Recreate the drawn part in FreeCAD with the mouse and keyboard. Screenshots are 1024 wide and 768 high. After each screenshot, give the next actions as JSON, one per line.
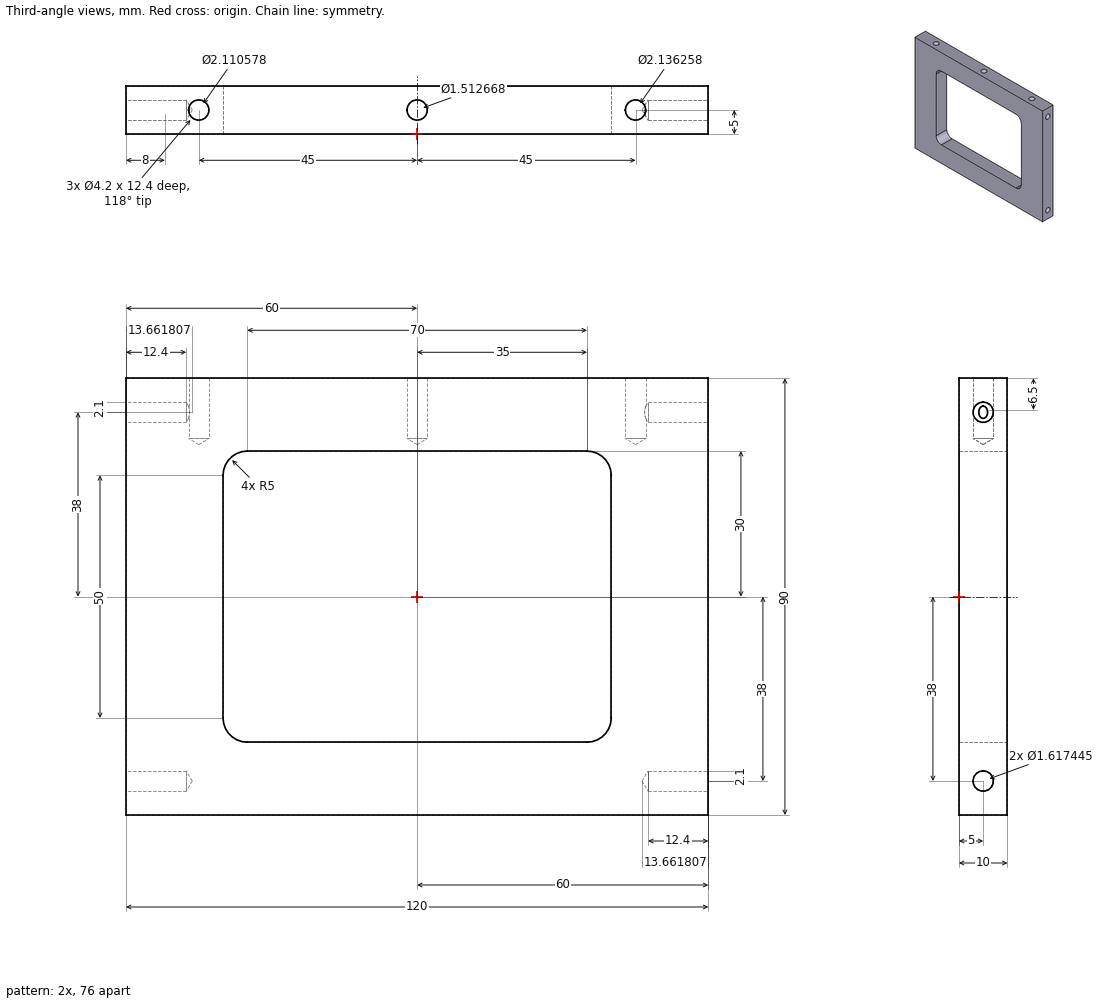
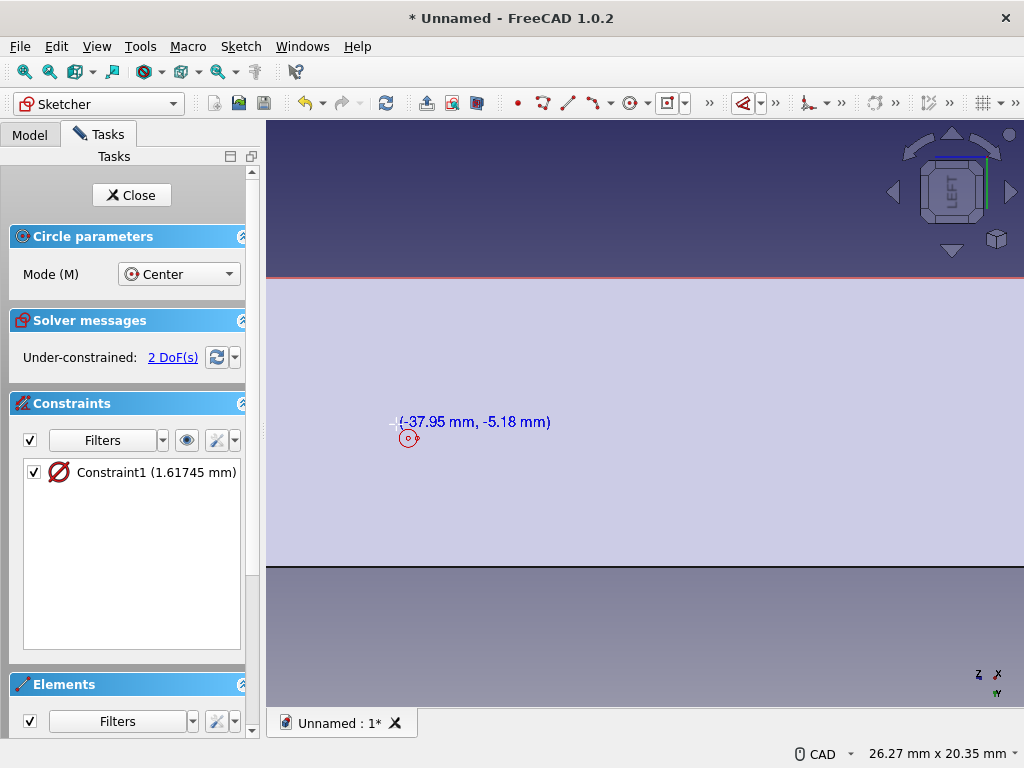
{"action": "scroll", "coordinate": [396, 424], "scroll_direction": "down", "scroll_amount": 9}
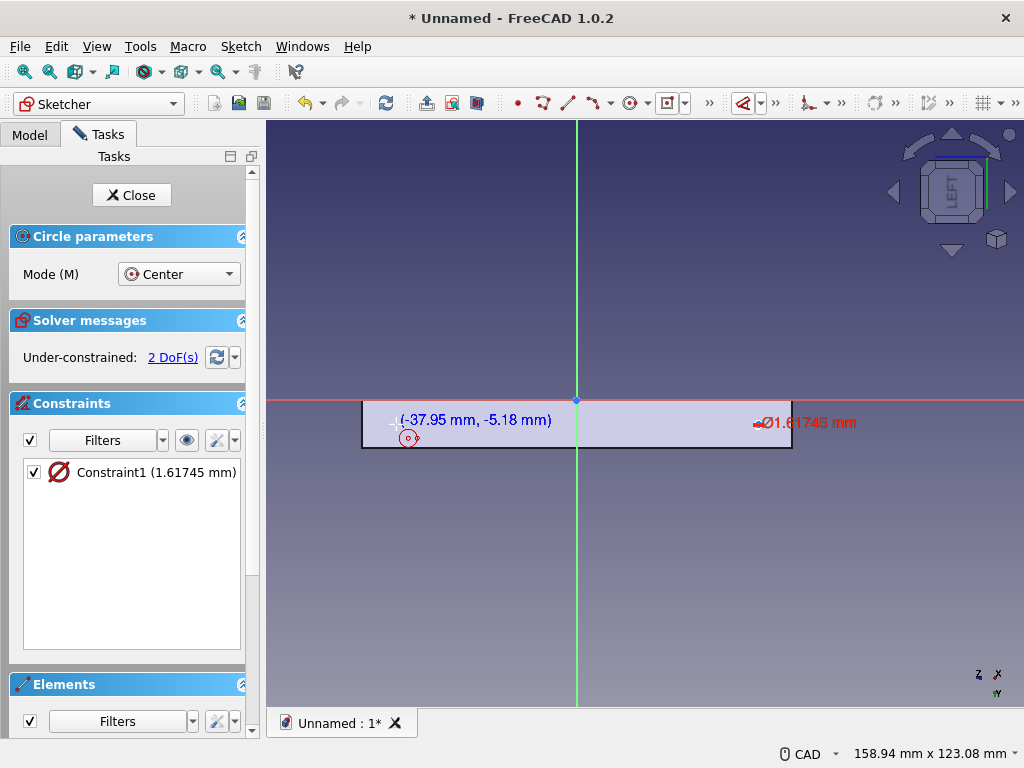
{"action": "left_click", "coordinate": [396, 424]}
{"action": "mouse_move", "coordinate": [398, 421]}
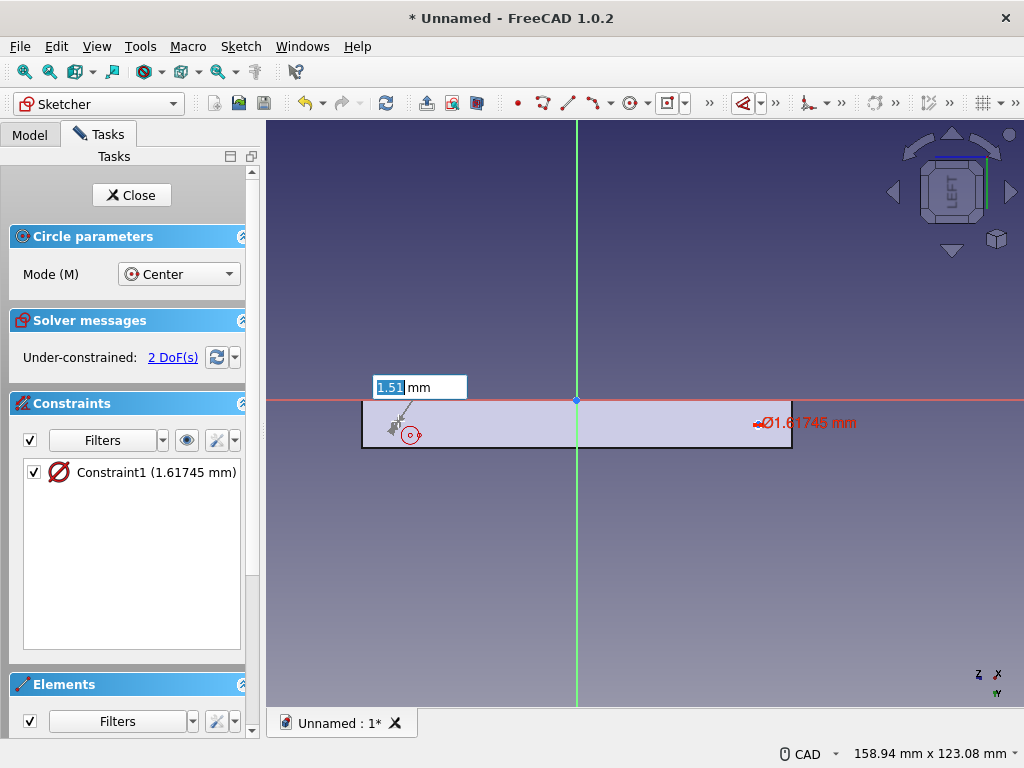
{"action": "type", "text": "1.617445"}
{"action": "key", "text": "Return"}
{"action": "key", "text": "Escape"}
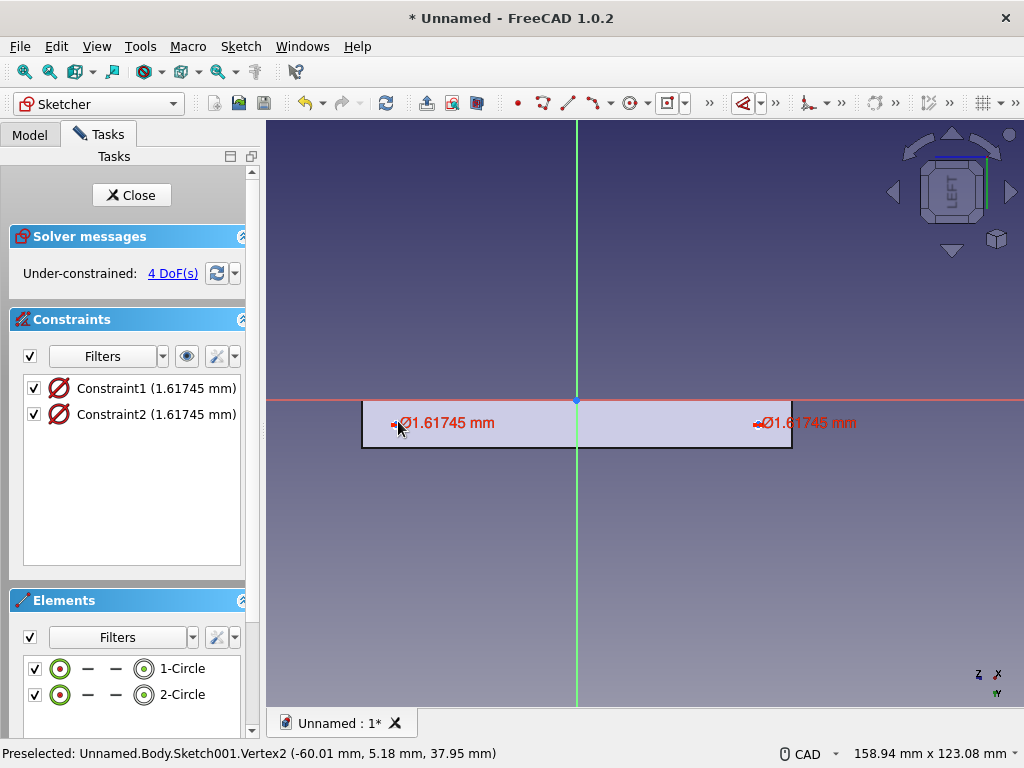
{"action": "left_click", "coordinate": [758, 425]}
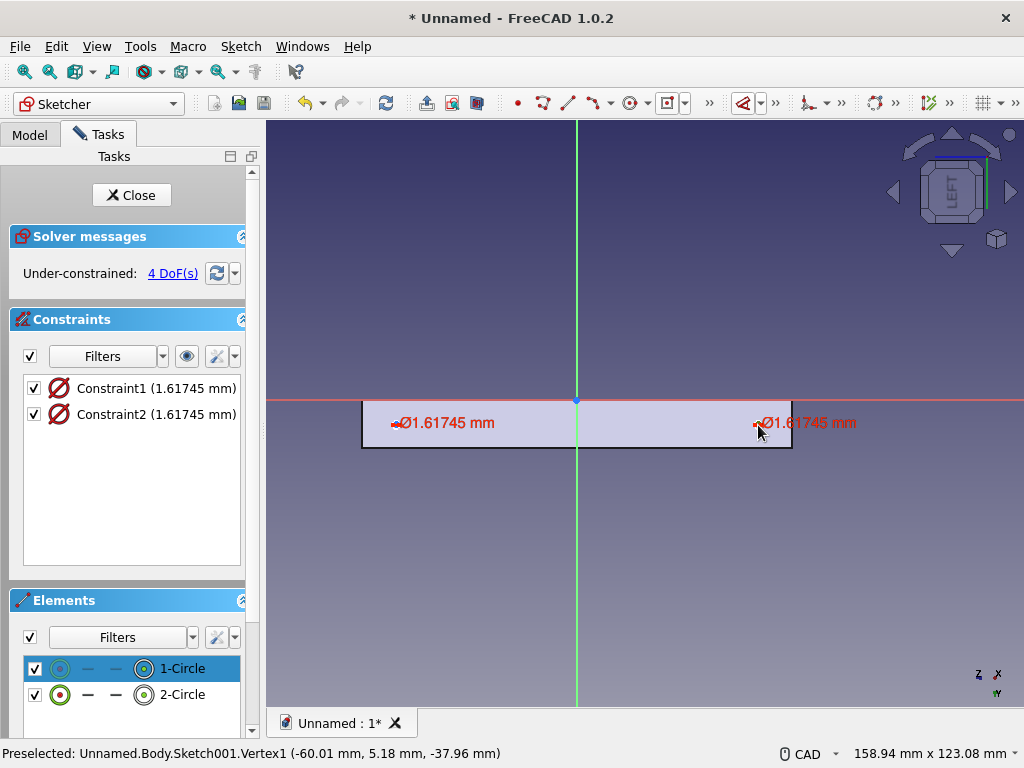
{"action": "left_click", "coordinate": [396, 425]}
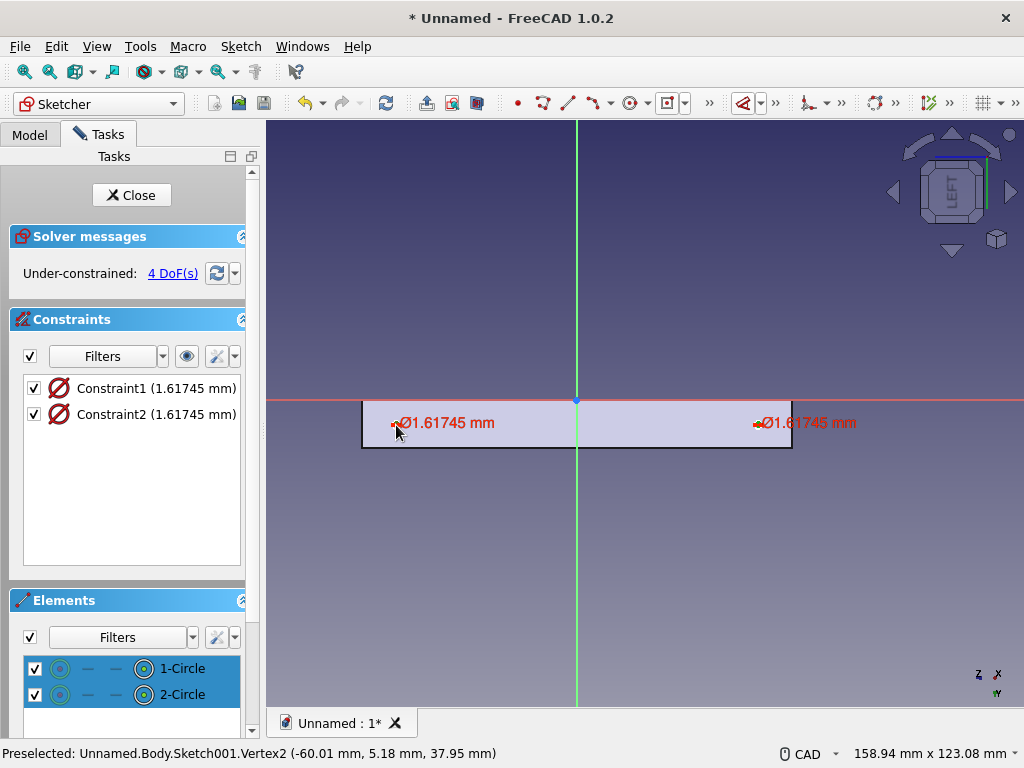
{"action": "left_click", "coordinate": [577, 641]}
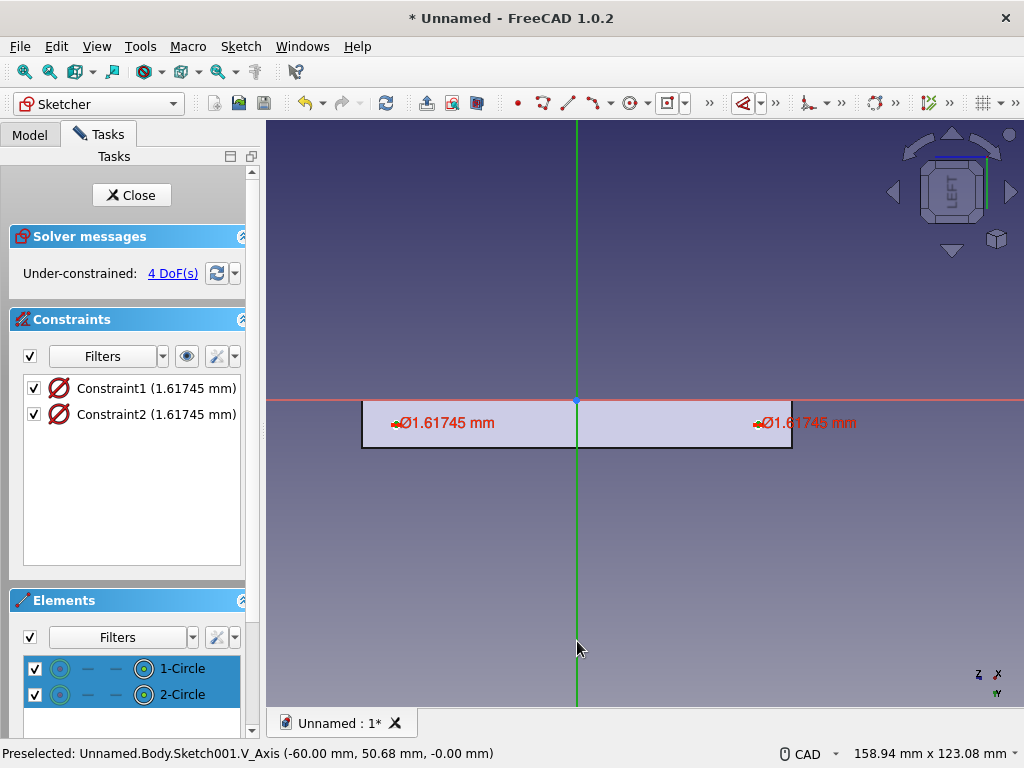
{"action": "key", "text": "s"}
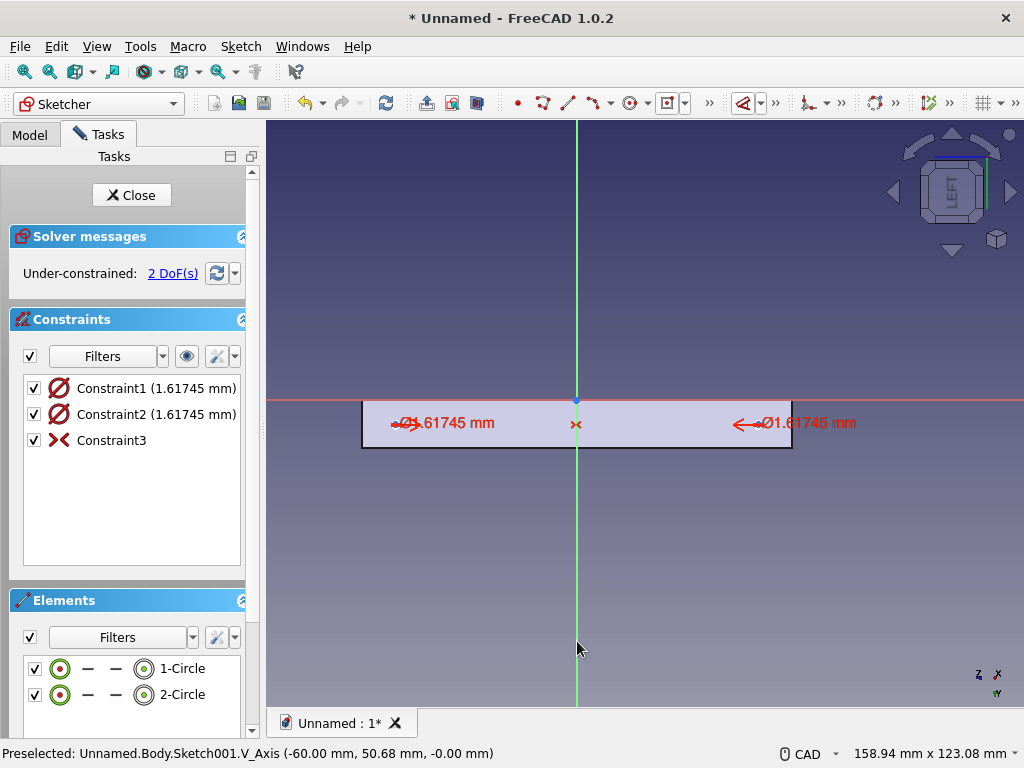
{"action": "left_click", "coordinate": [742, 104]}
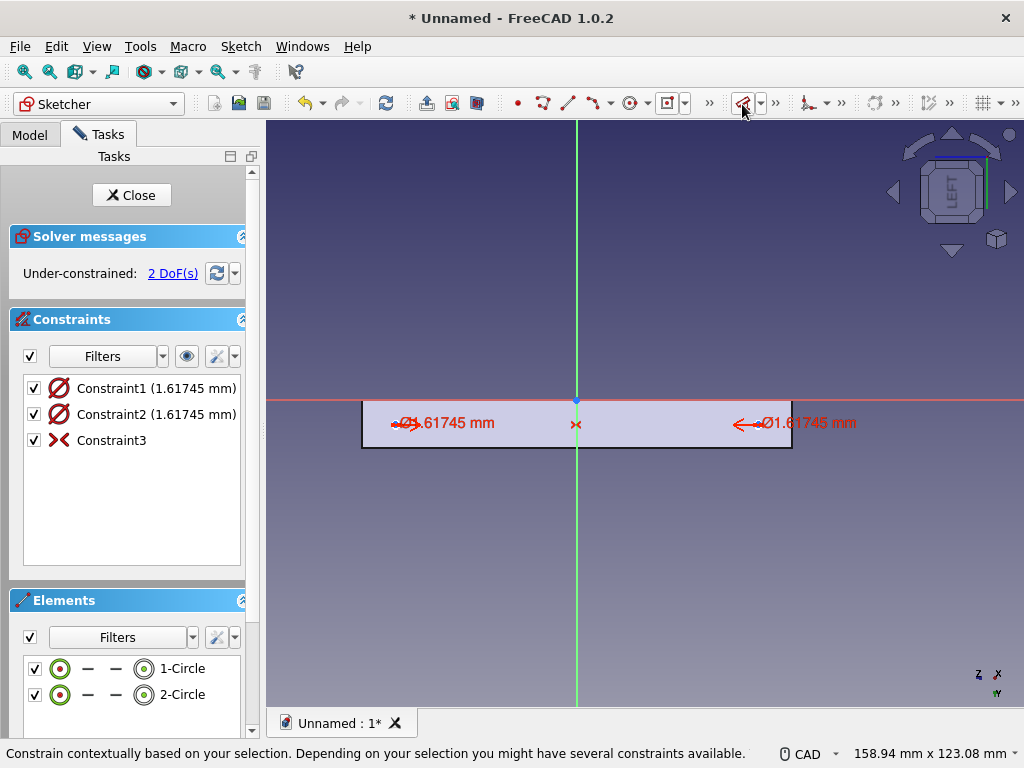
{"action": "scroll", "coordinate": [758, 425], "scroll_direction": "up", "scroll_amount": 3}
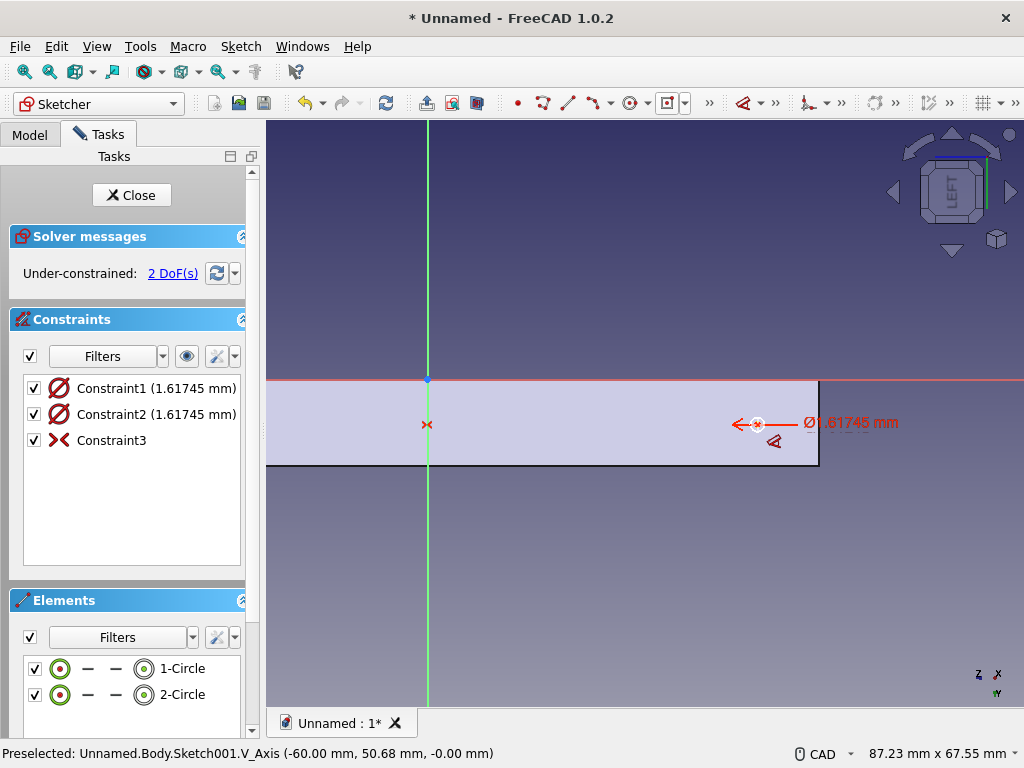
{"action": "left_click", "coordinate": [757, 425]}
{"action": "left_click", "coordinate": [791, 402]}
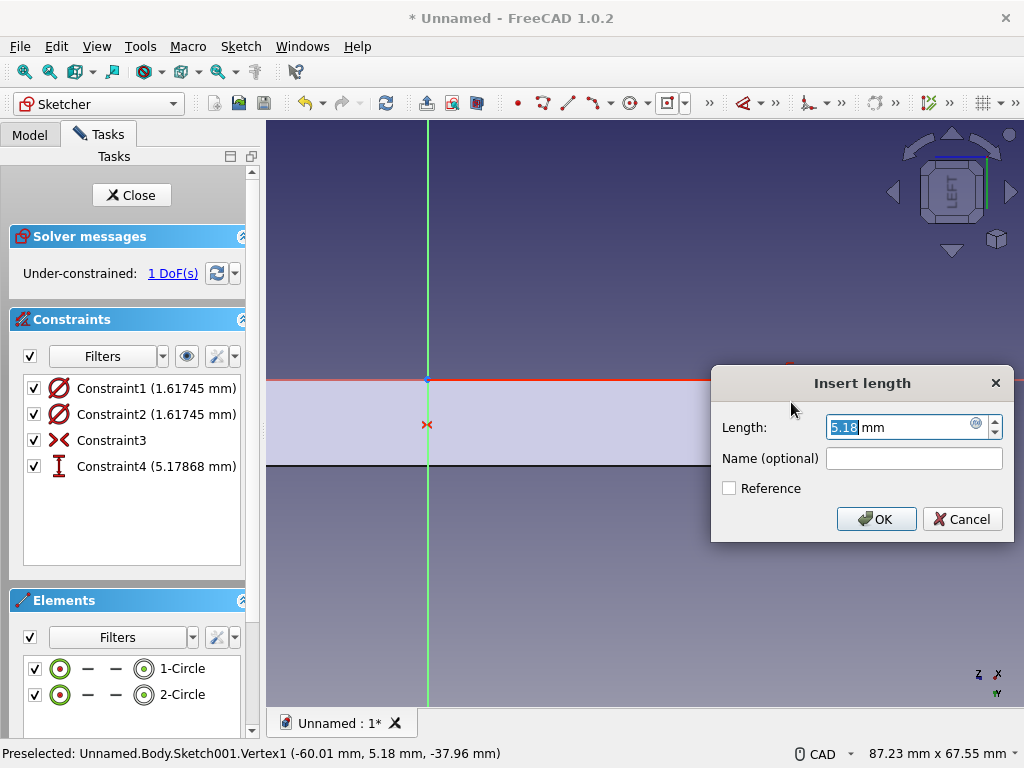
{"action": "type", "text": "5"}
{"action": "key", "text": "Return"}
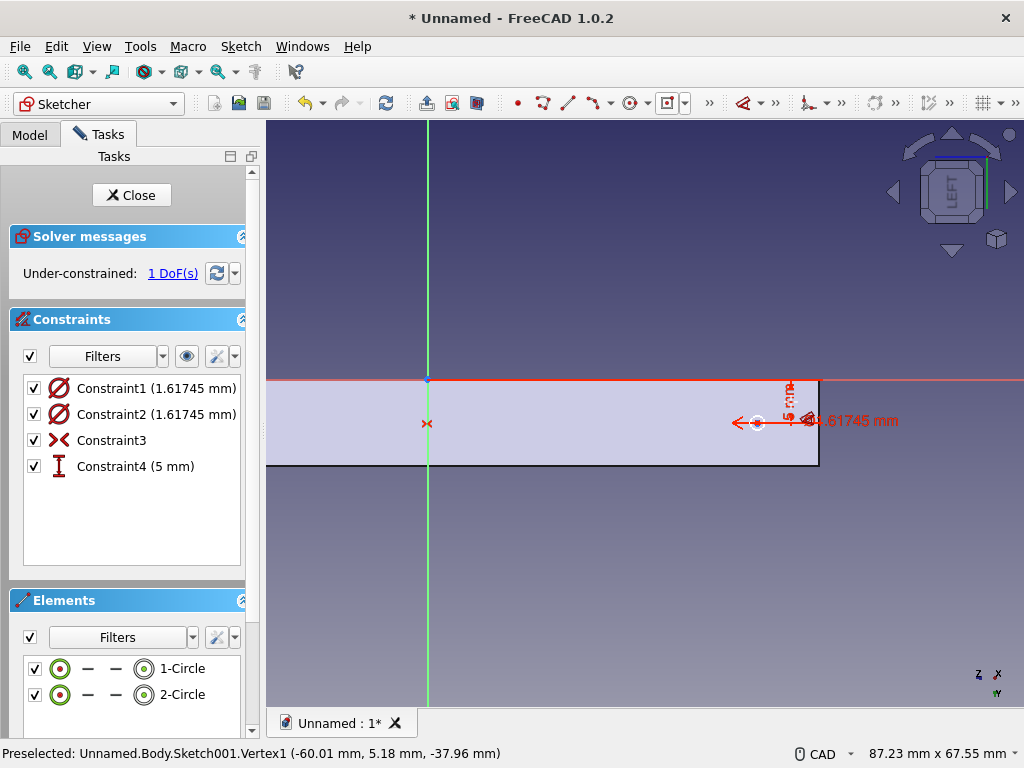
{"action": "left_click", "coordinate": [757, 423]}
{"action": "left_click", "coordinate": [593, 346]}